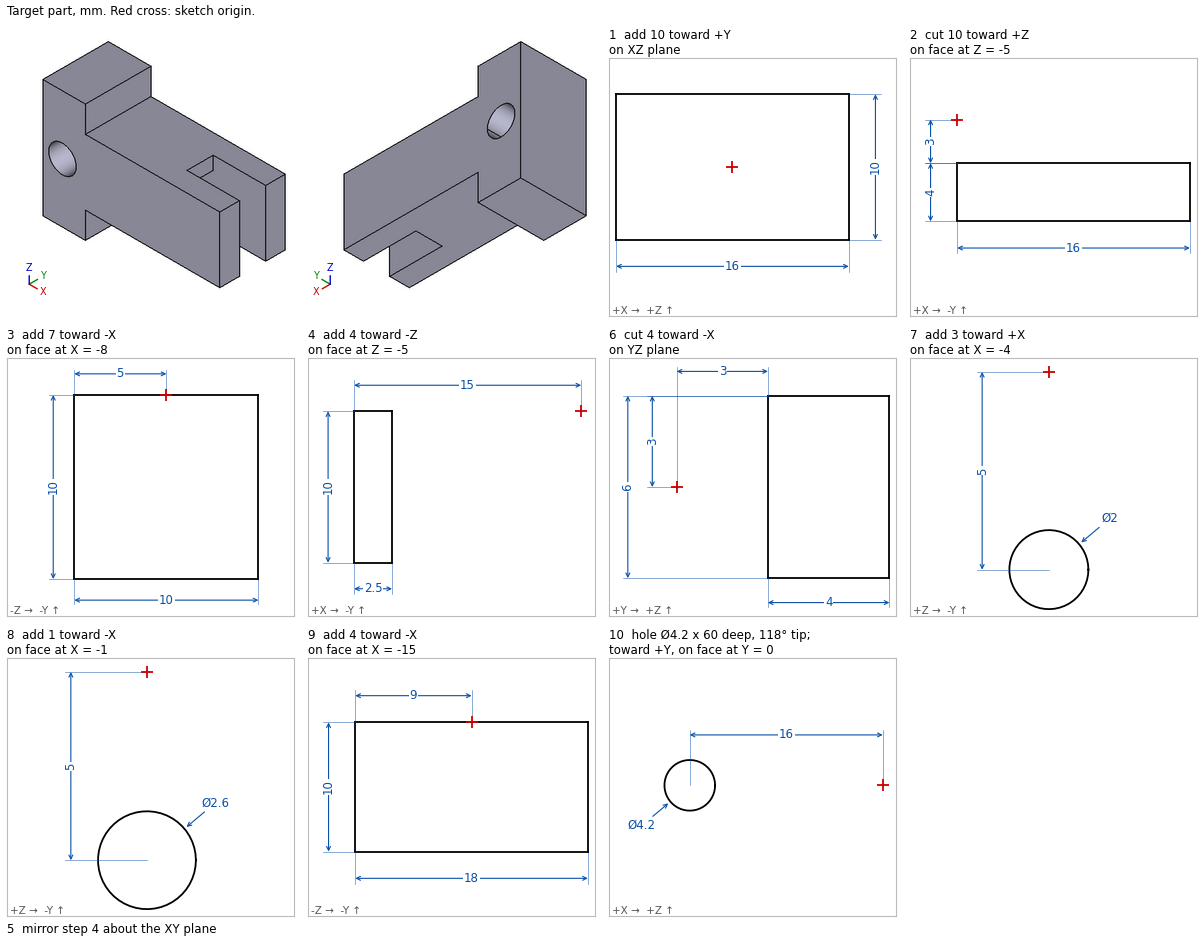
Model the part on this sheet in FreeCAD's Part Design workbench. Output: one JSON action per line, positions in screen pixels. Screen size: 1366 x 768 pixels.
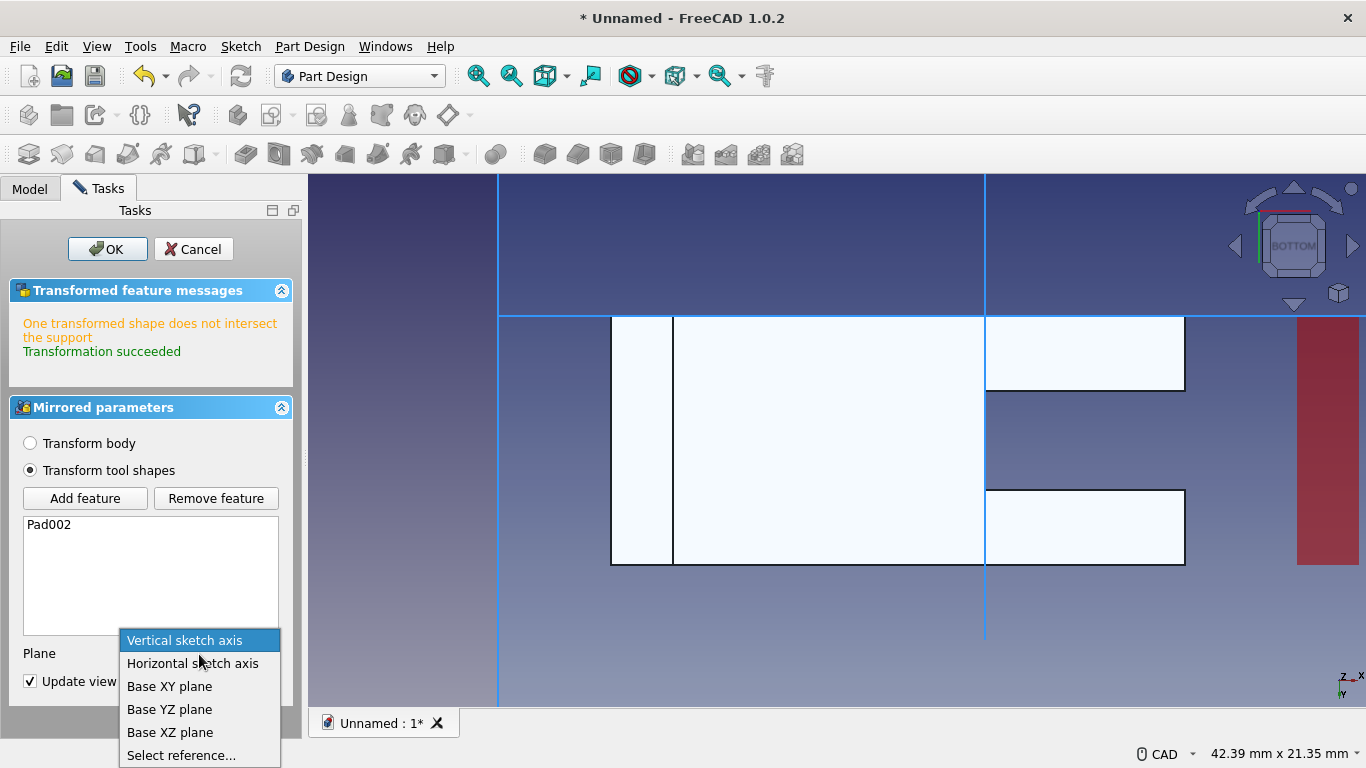
{"action": "left_click", "coordinate": [198, 686]}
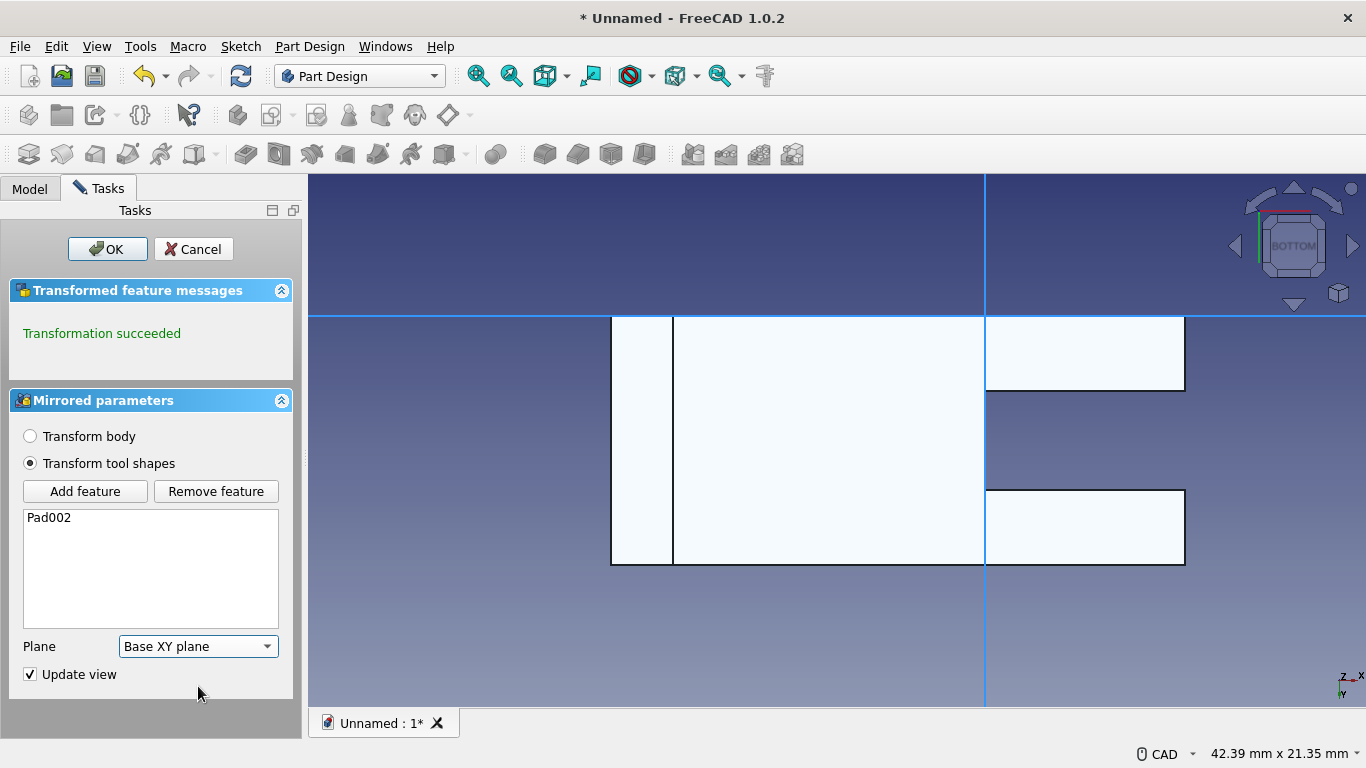
{"action": "left_click", "coordinate": [108, 249]}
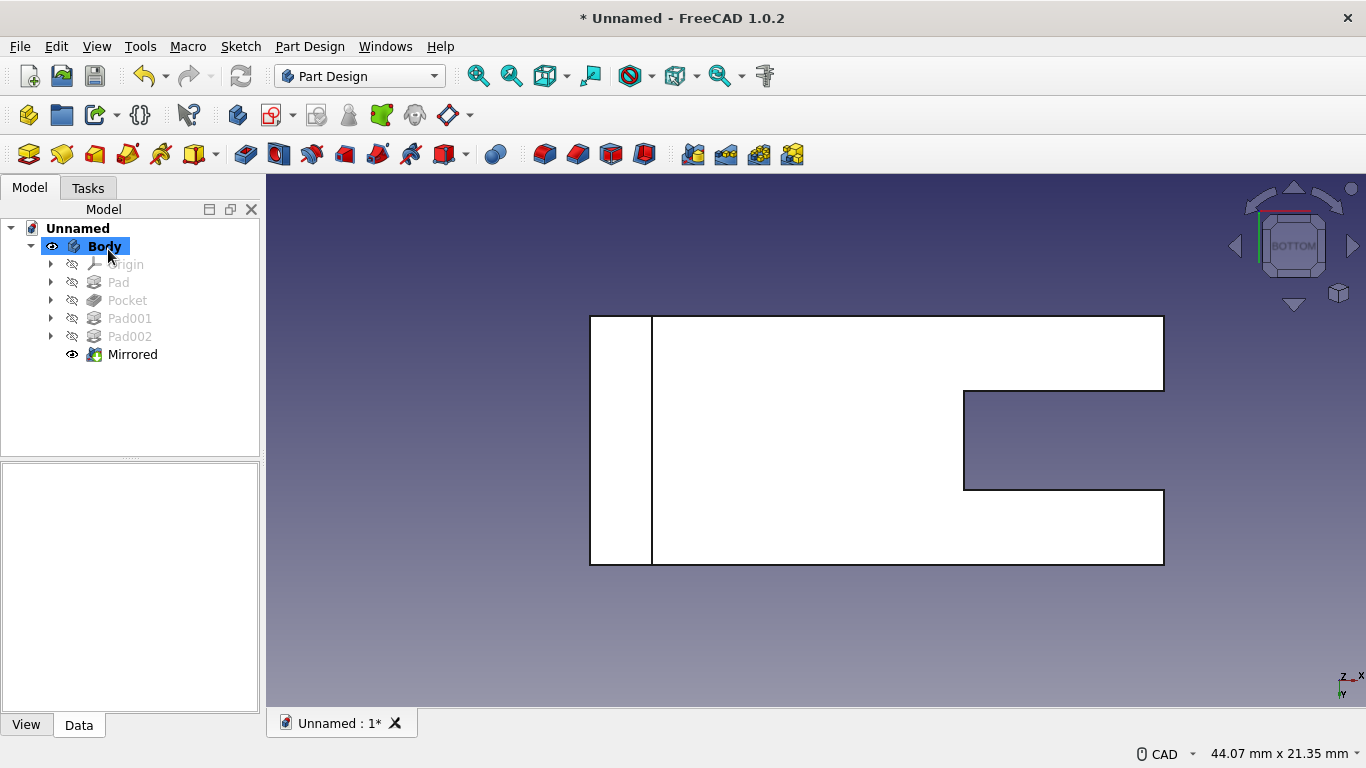
{"action": "left_click", "coordinate": [270, 116]}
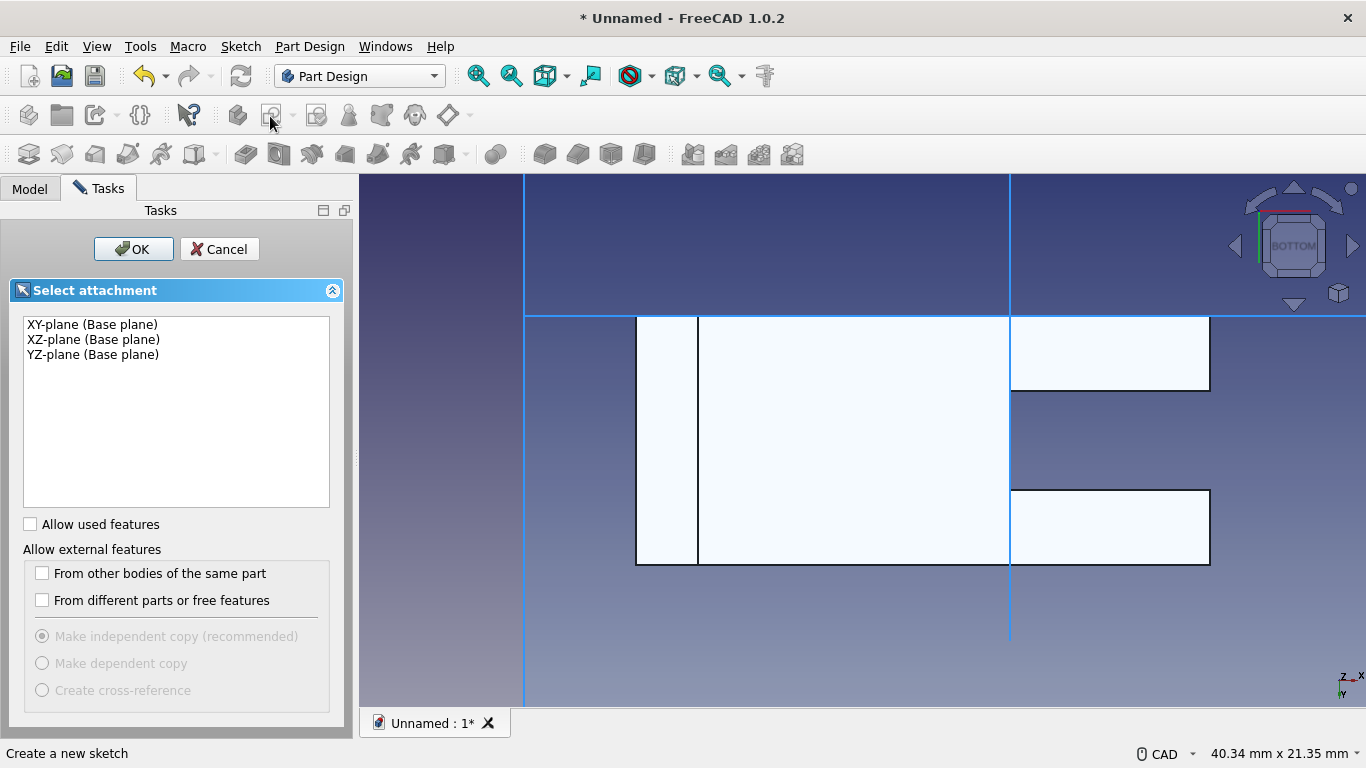
{"action": "left_click", "coordinate": [84, 354]}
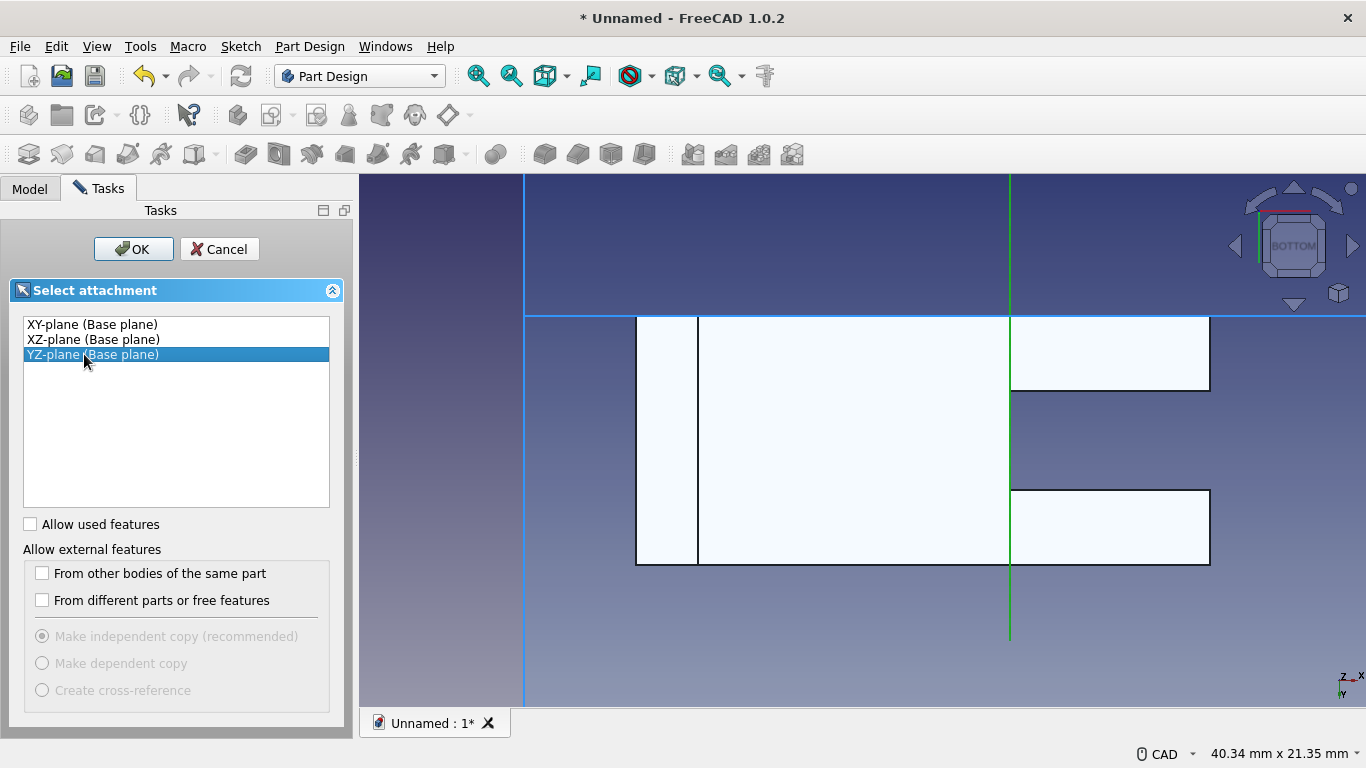
{"action": "left_click", "coordinate": [134, 249]}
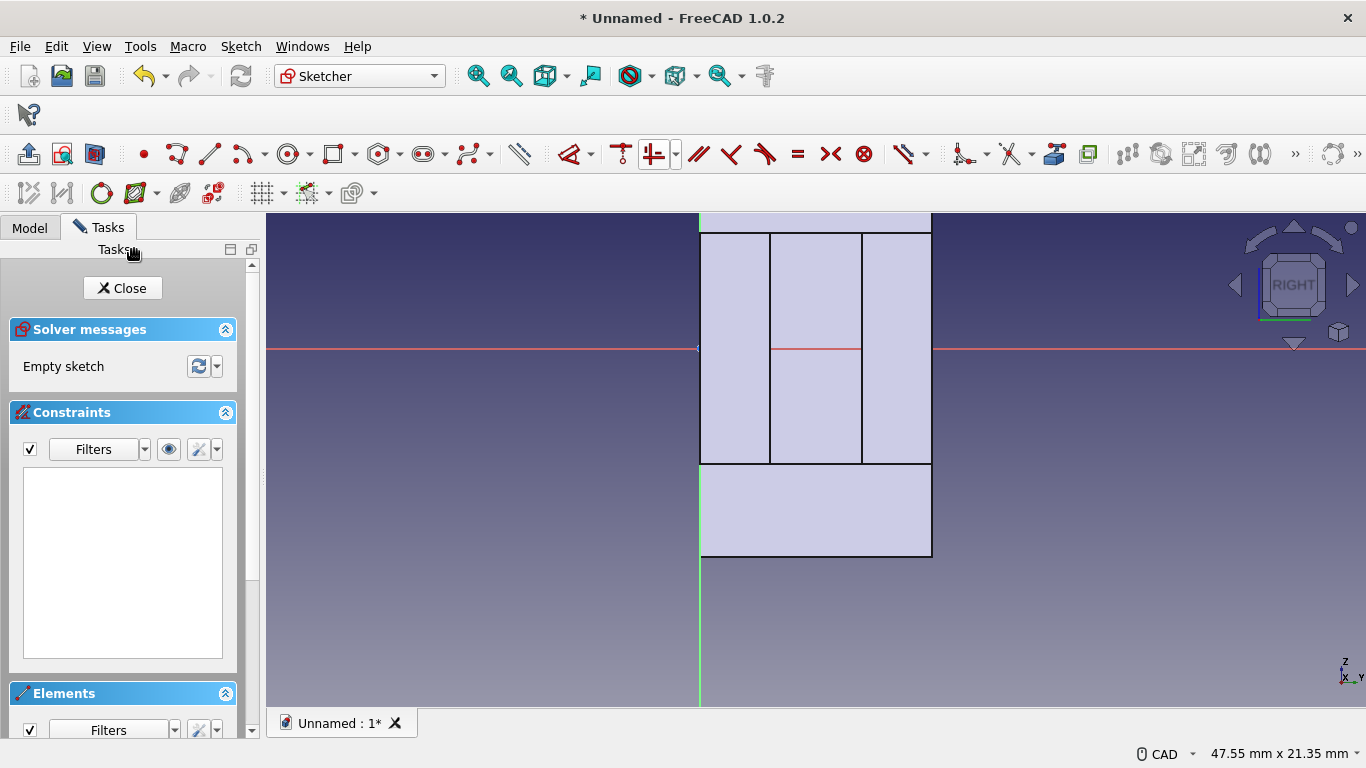
{"action": "left_click", "coordinate": [95, 154]}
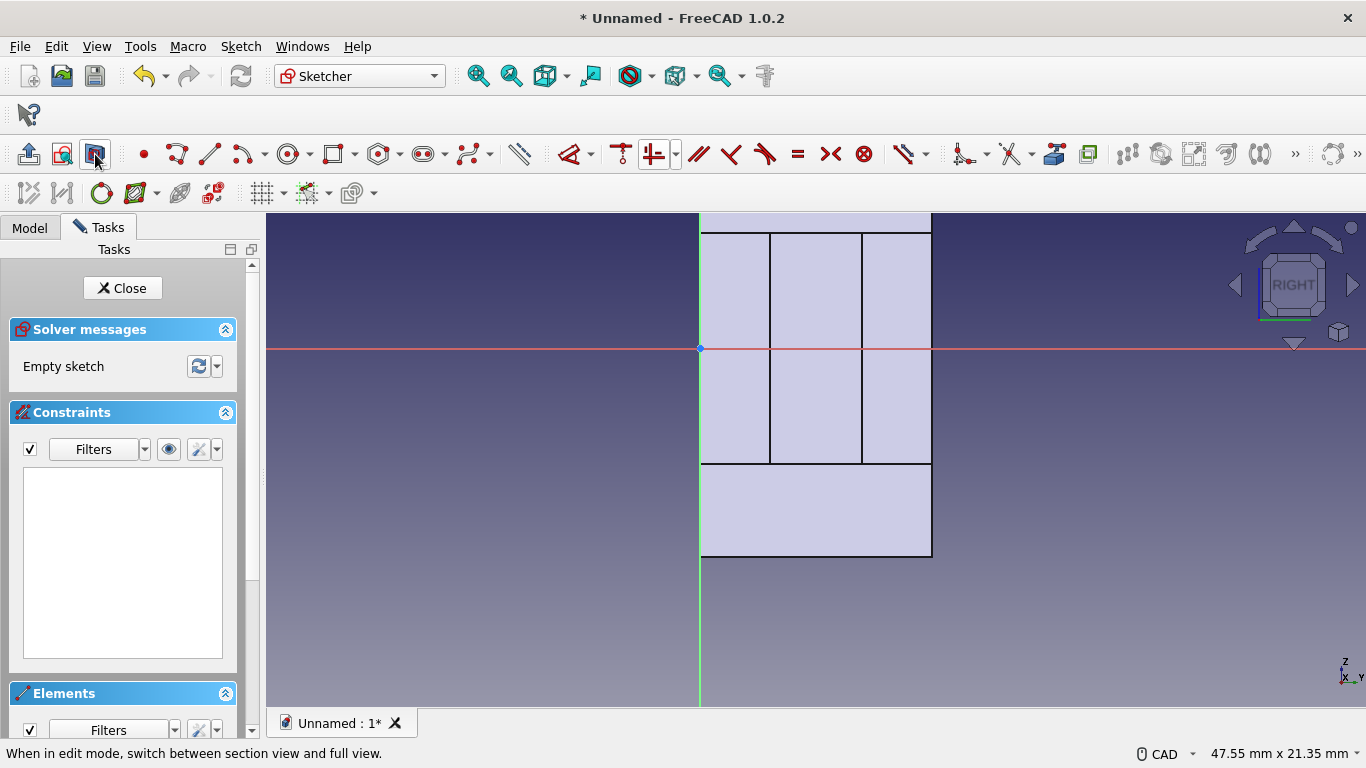
{"action": "scroll", "coordinate": [809, 258], "scroll_direction": "up", "scroll_amount": 4}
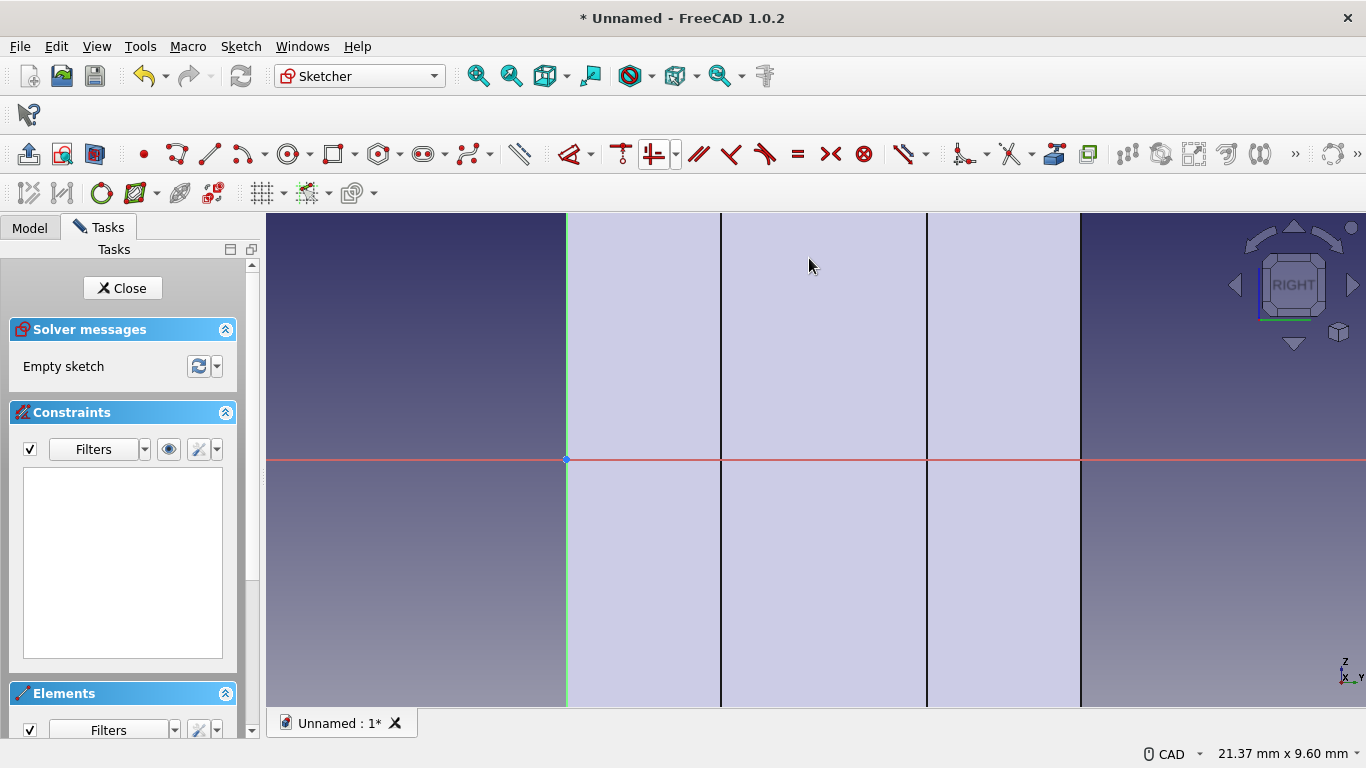
{"action": "left_click", "coordinate": [332, 154]}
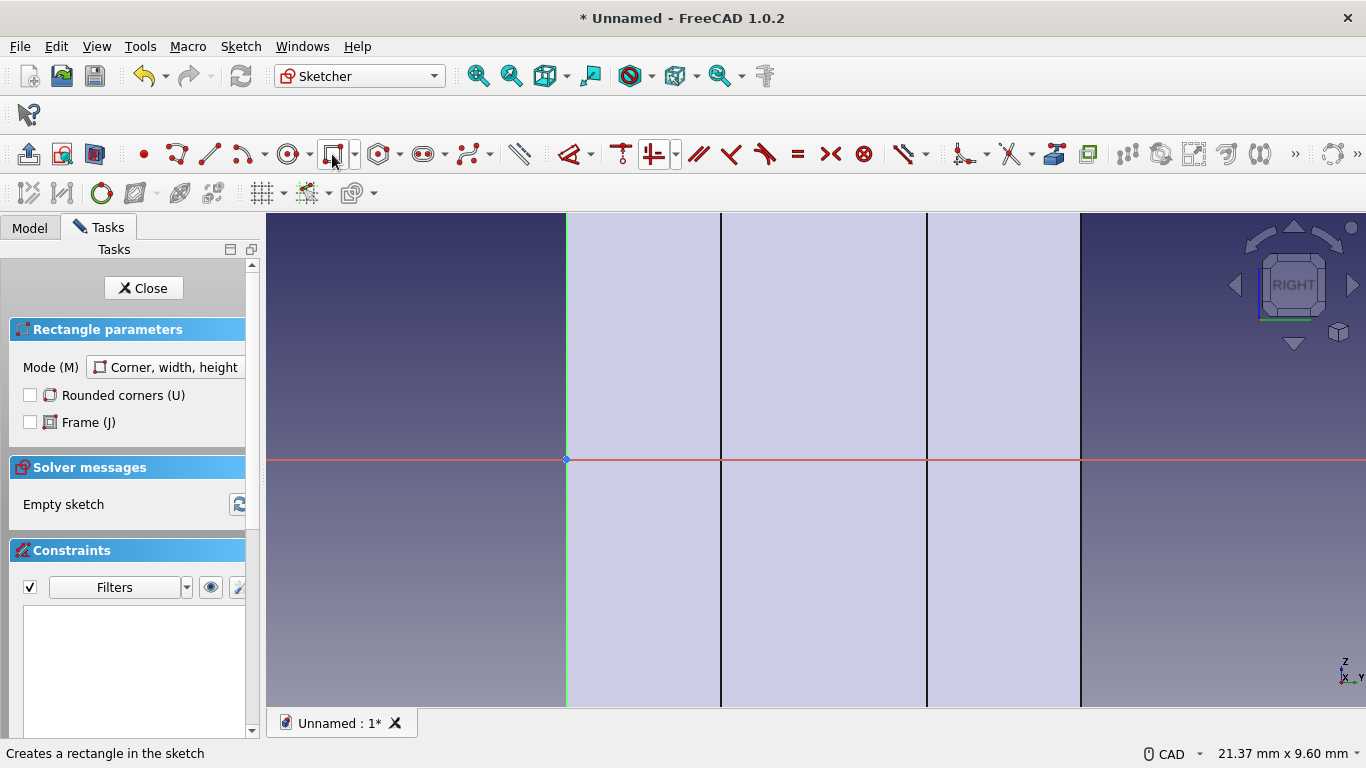
{"action": "left_click", "coordinate": [721, 305]}
{"action": "left_click", "coordinate": [927, 614]}
{"action": "key", "text": "Escape"}